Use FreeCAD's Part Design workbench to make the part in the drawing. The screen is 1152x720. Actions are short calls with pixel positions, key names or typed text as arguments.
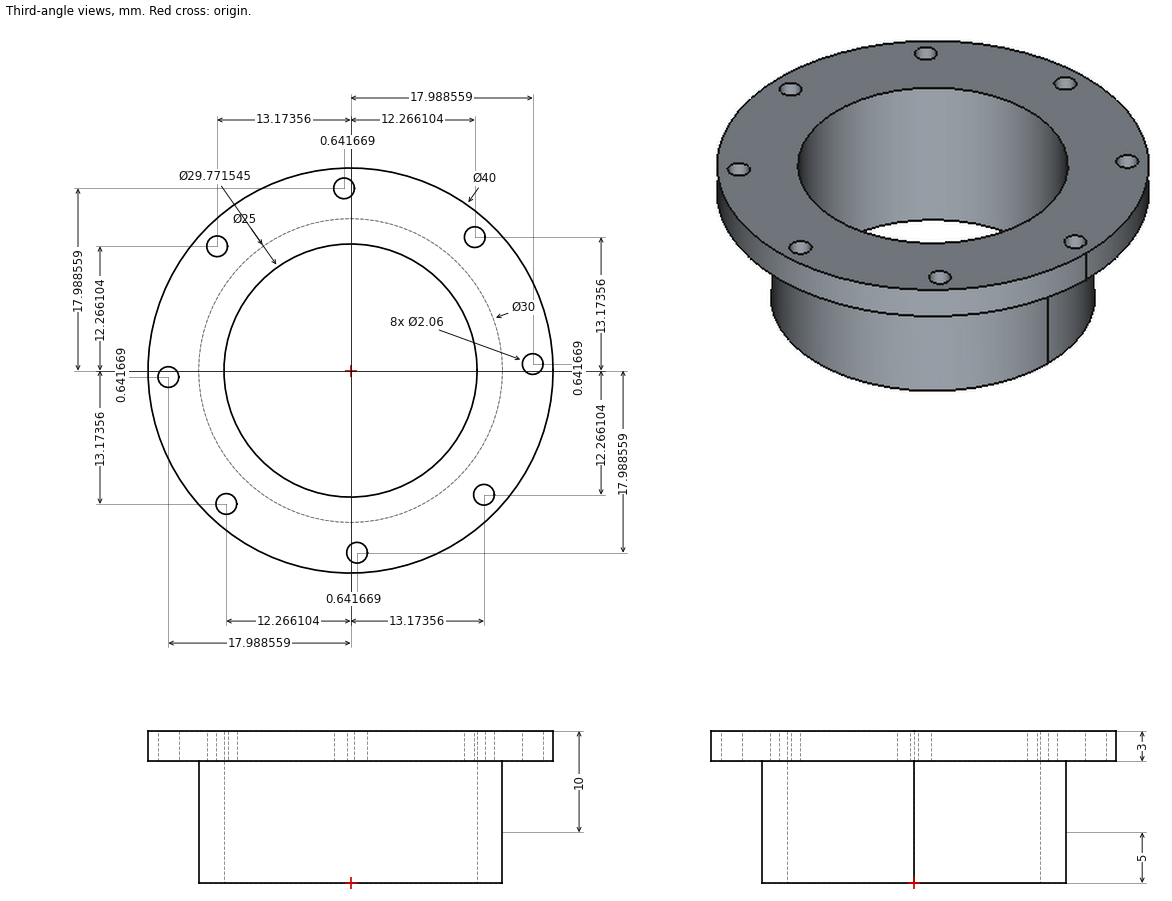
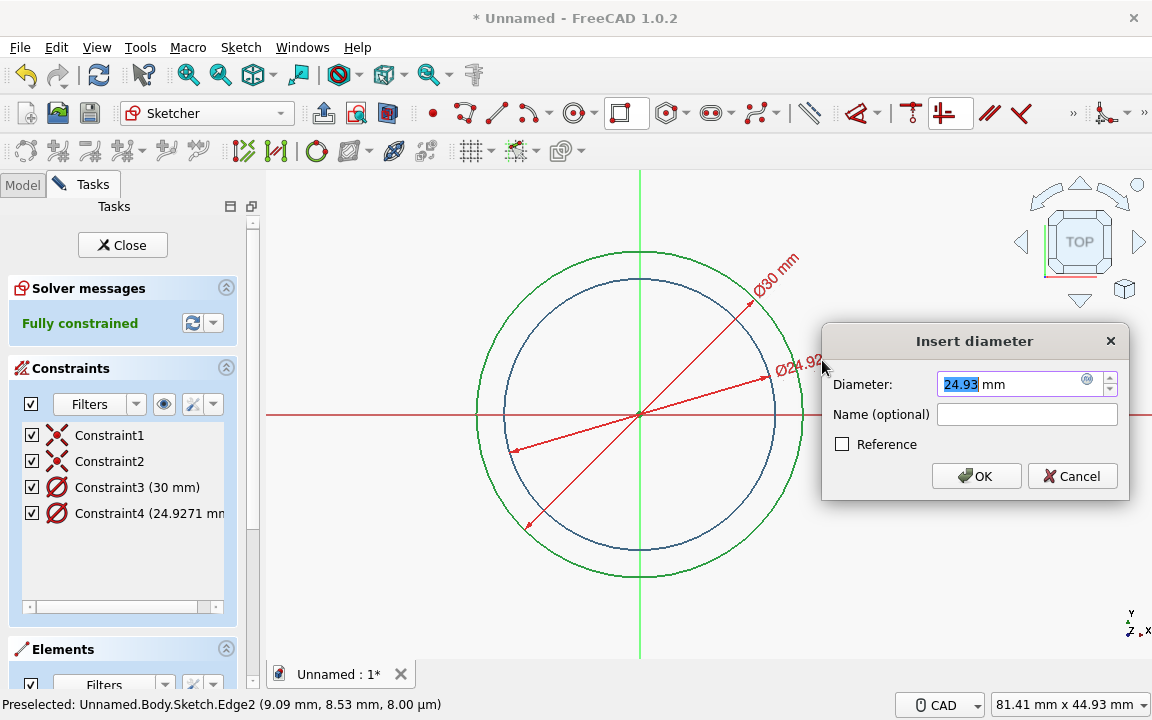
text(25)
key(Return)
key(Escape)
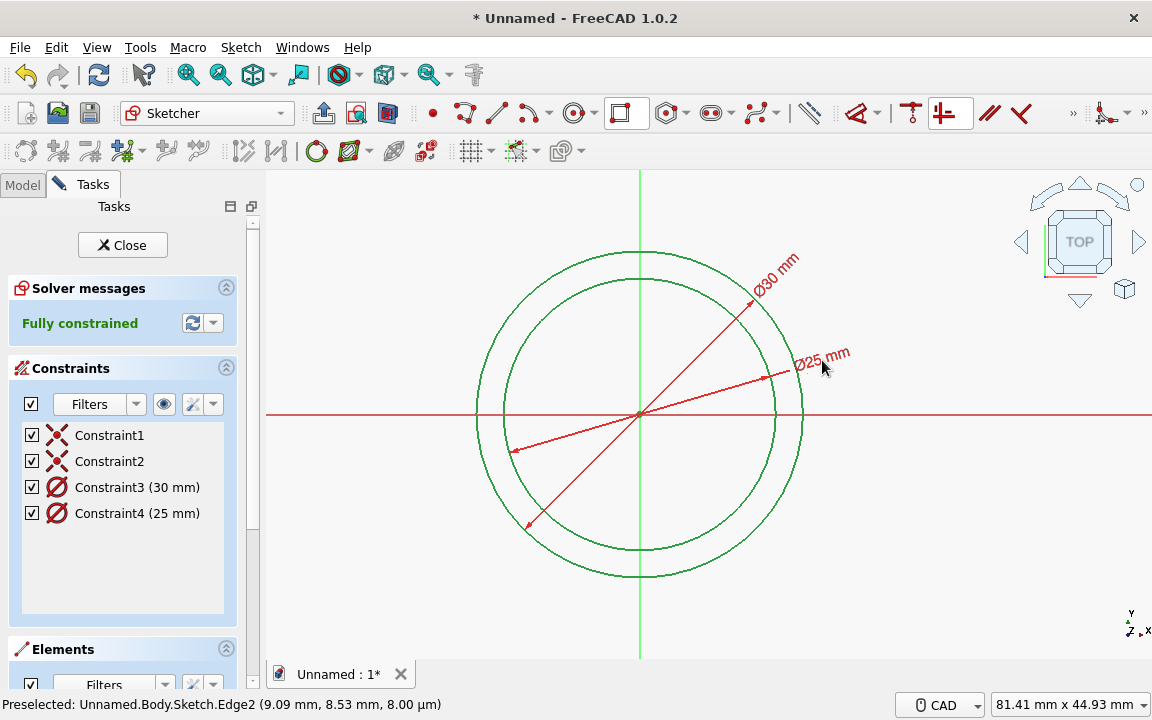
click(123, 245)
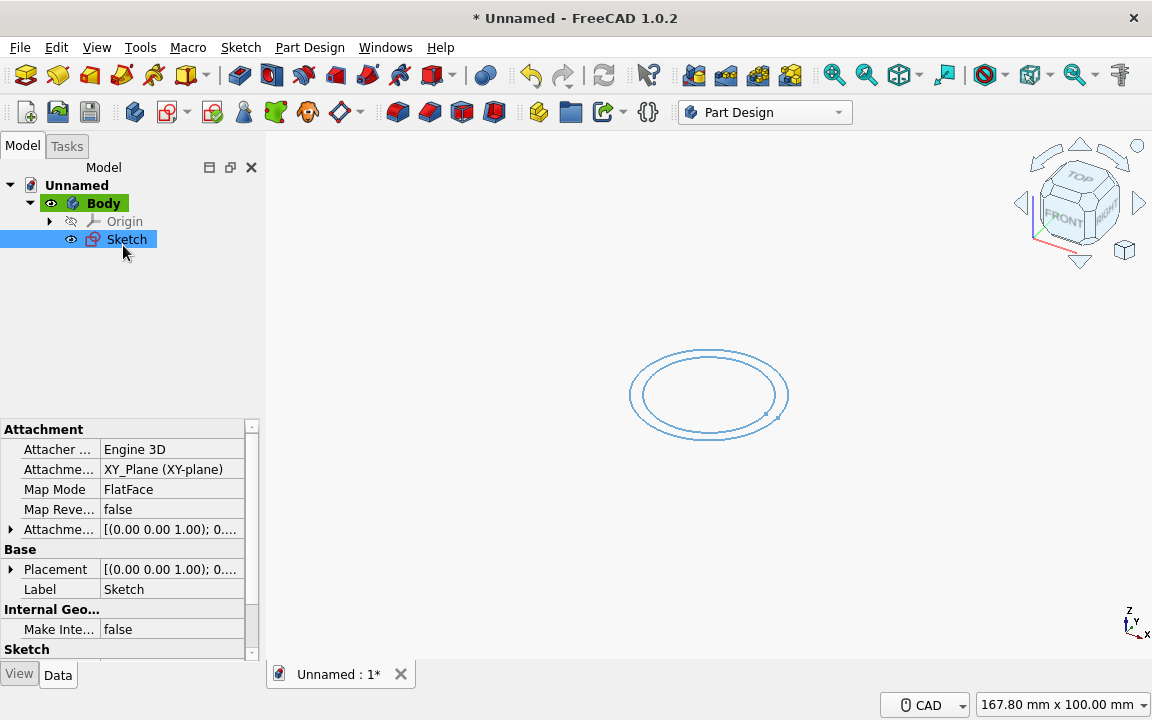
click(26, 76)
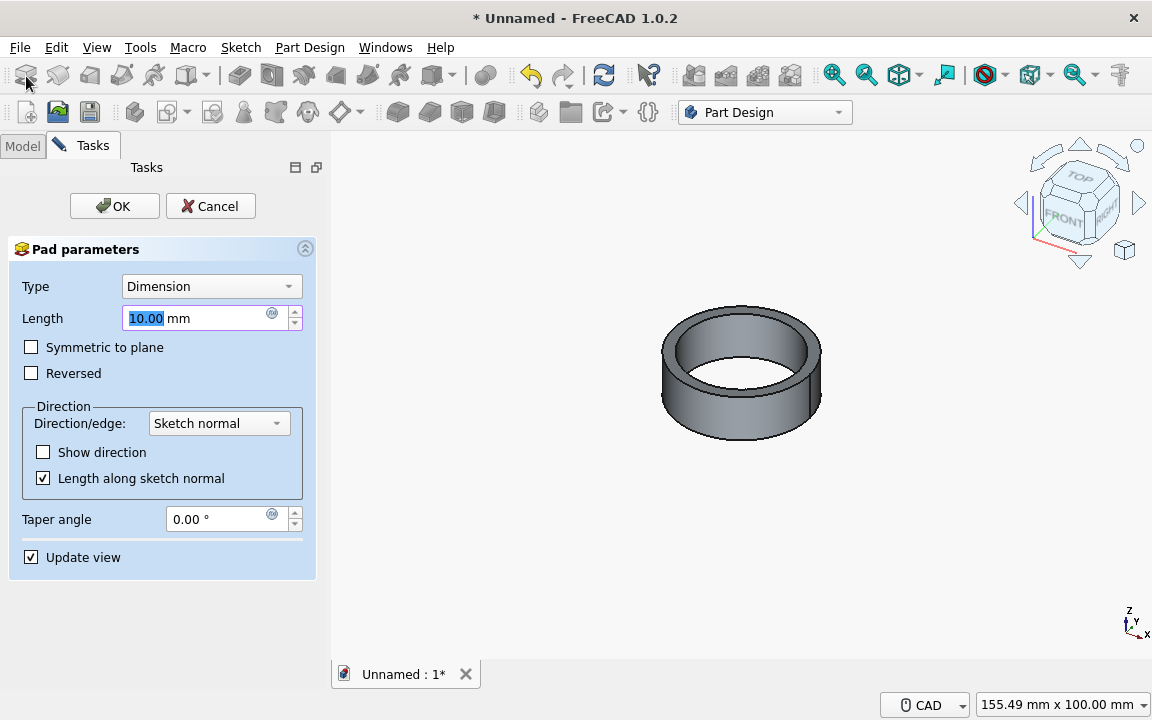
text(5)
key(Tab)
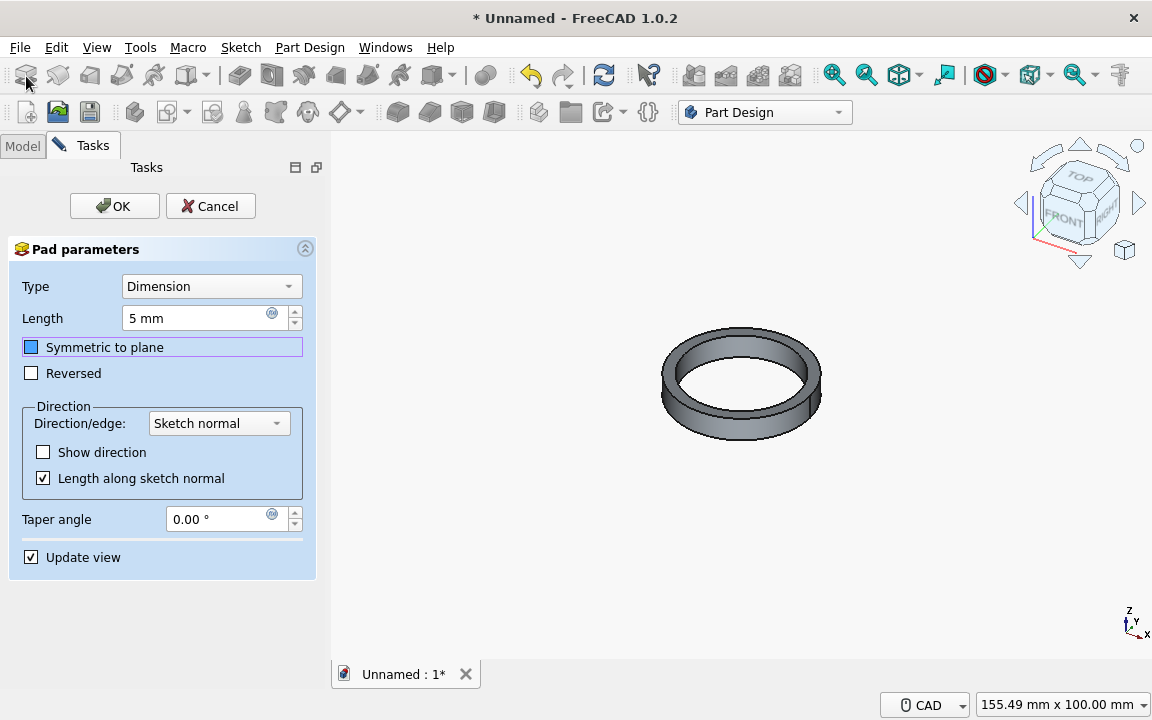
click(115, 206)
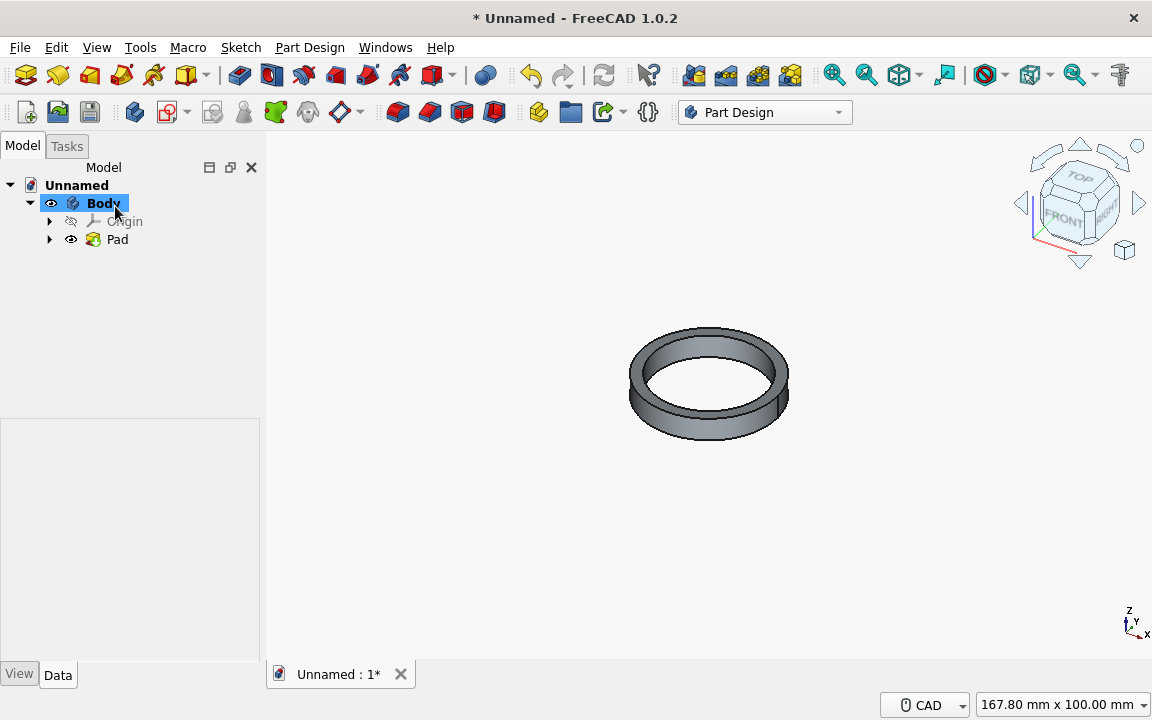
click(836, 76)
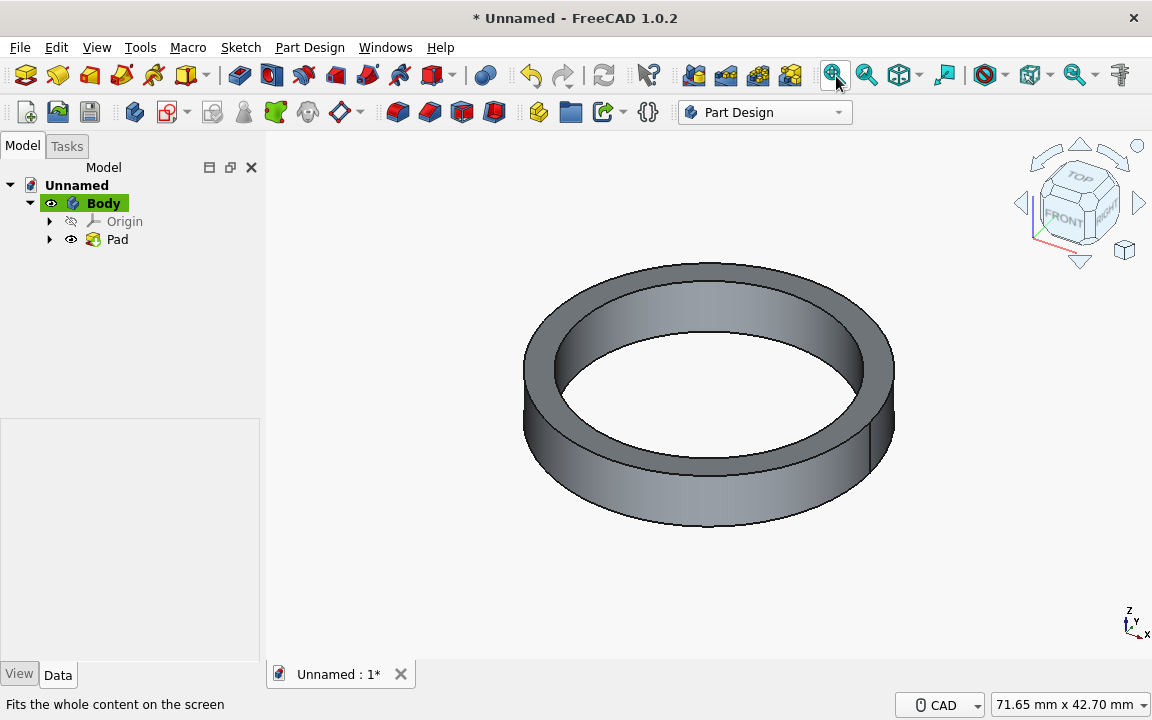
click(583, 432)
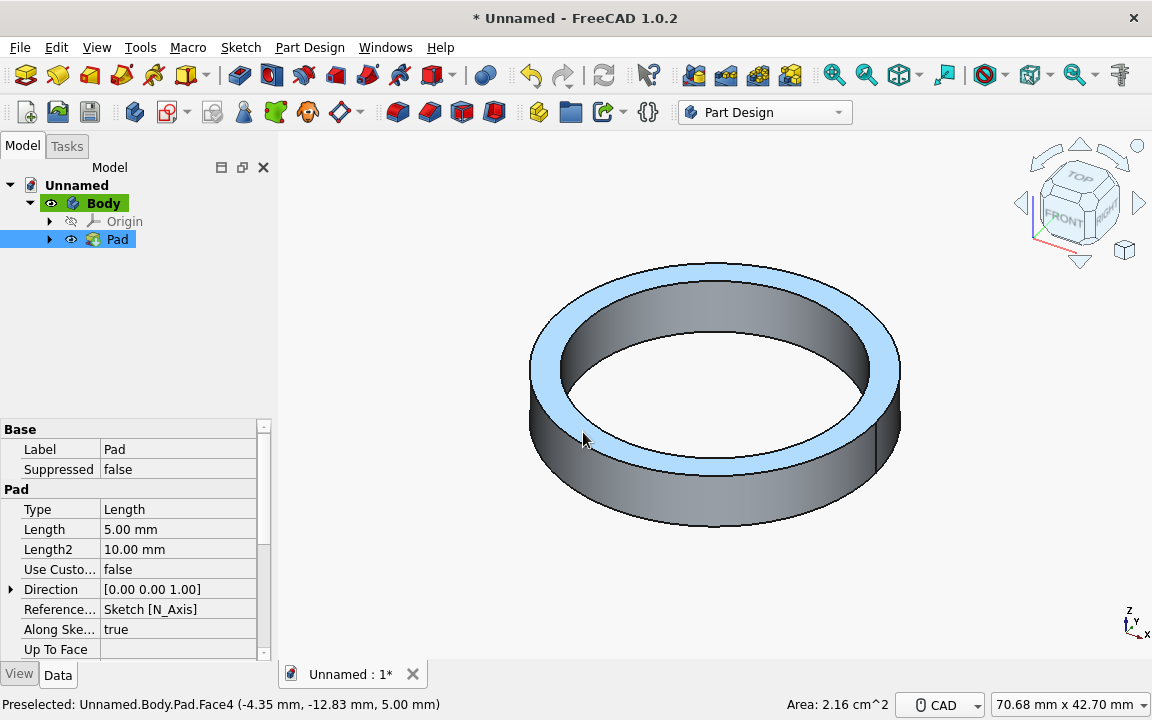
click(168, 112)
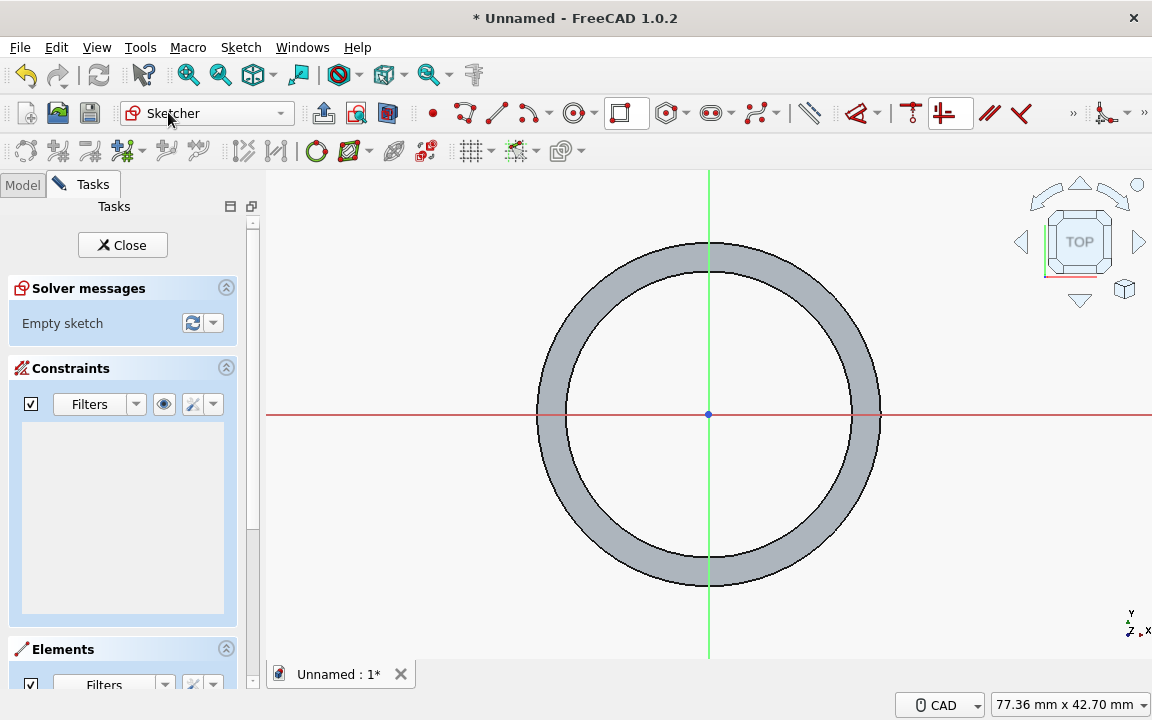
key(g)
key(c)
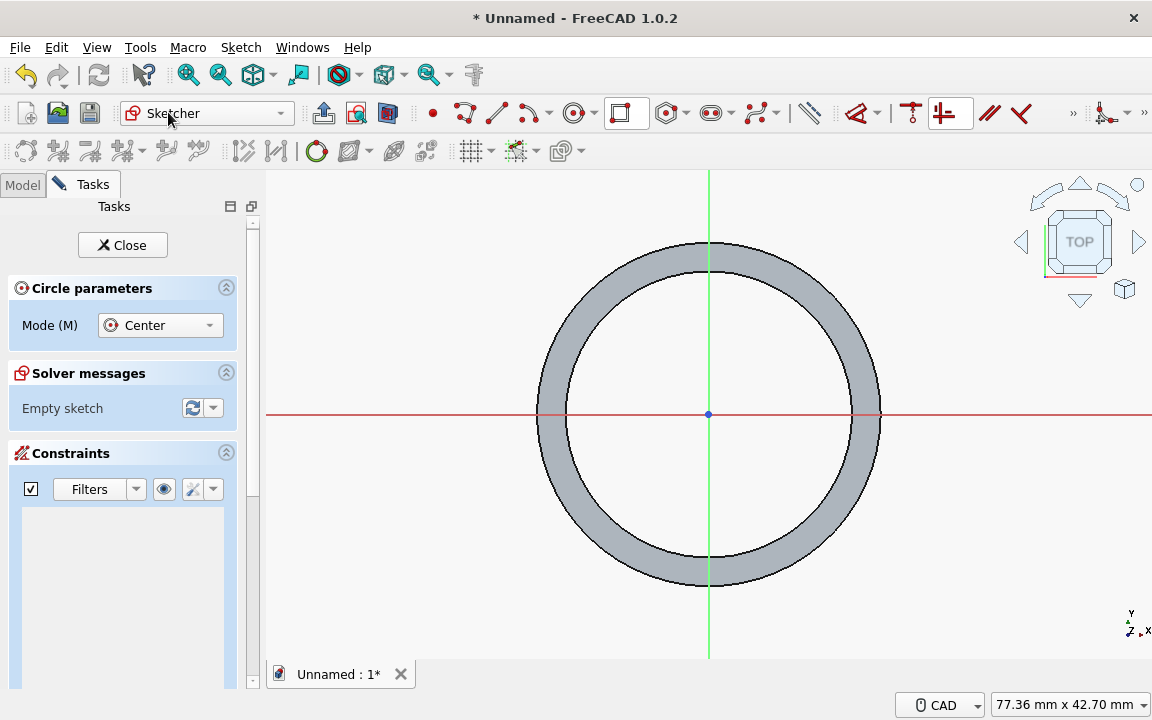
click(709, 414)
click(830, 293)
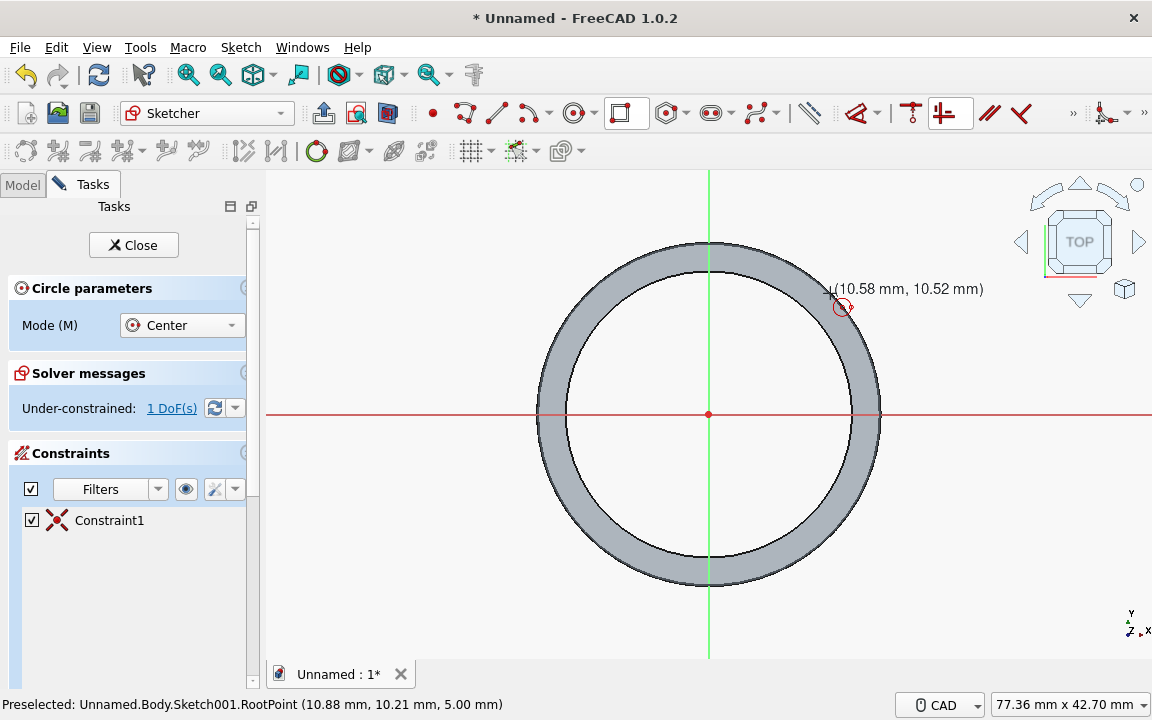
click(709, 414)
click(810, 313)
key(Escape)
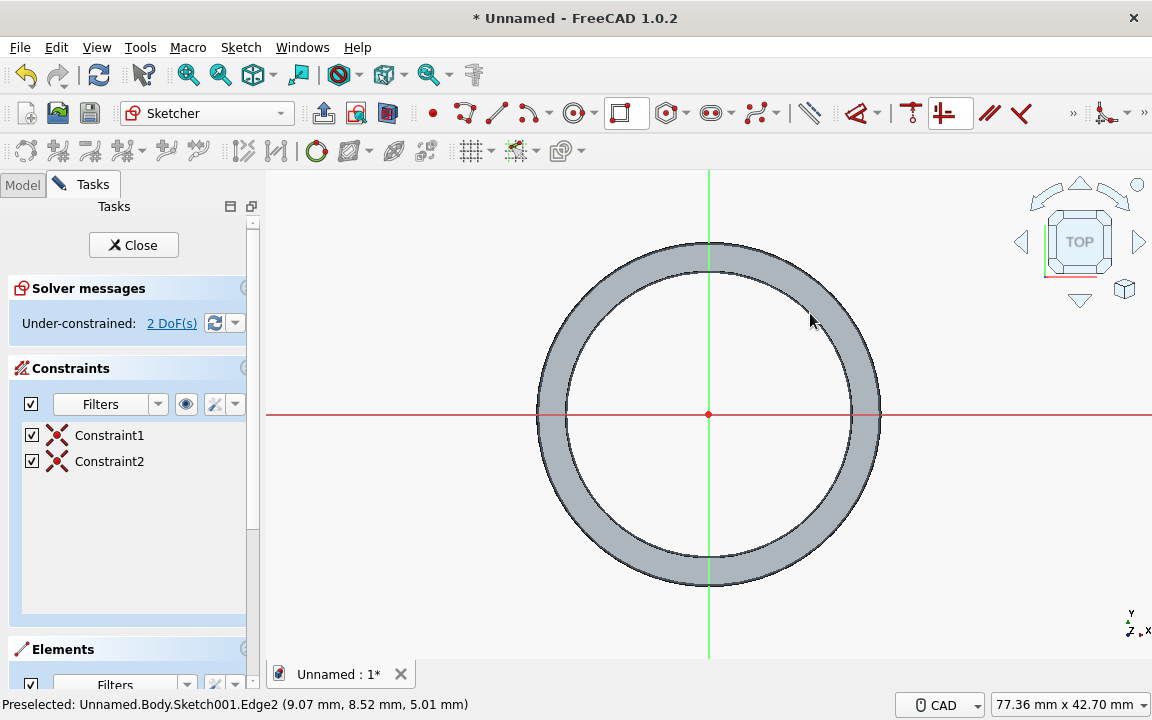
key(d)